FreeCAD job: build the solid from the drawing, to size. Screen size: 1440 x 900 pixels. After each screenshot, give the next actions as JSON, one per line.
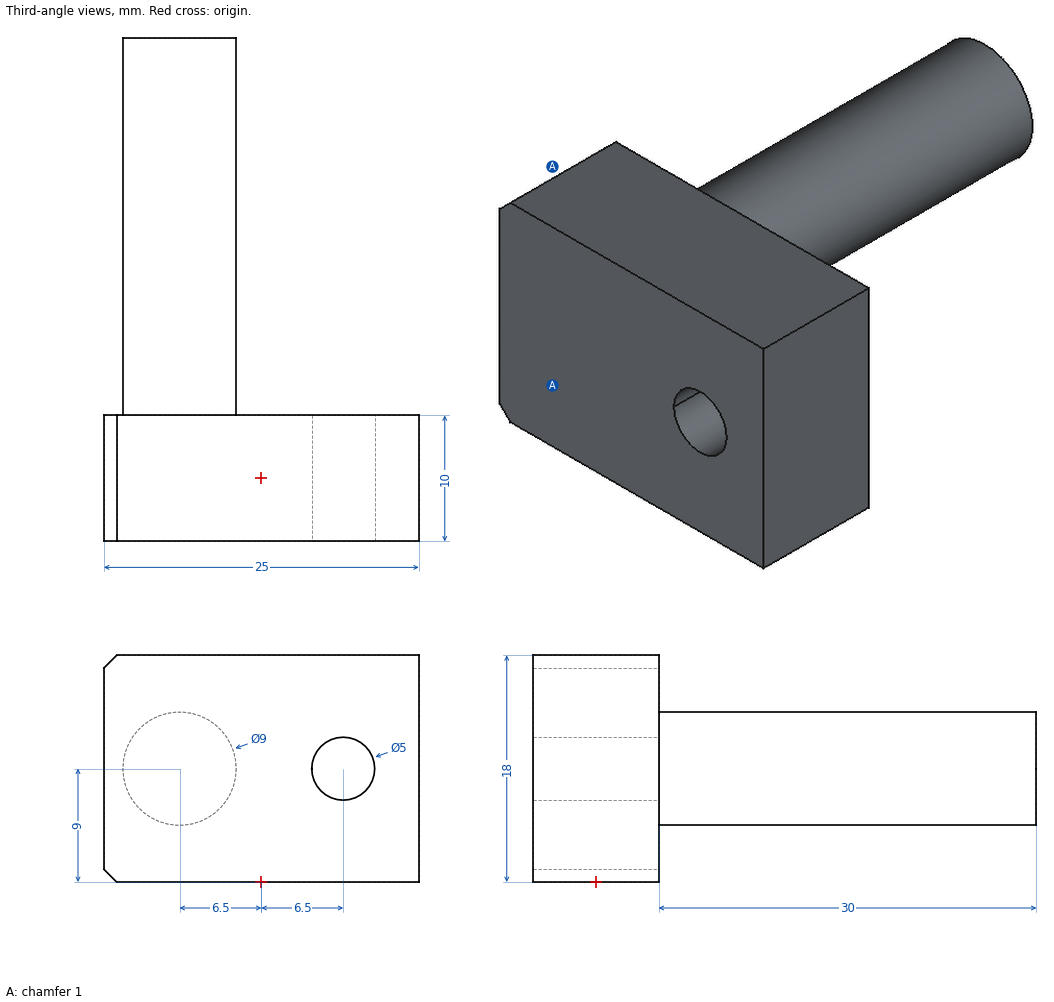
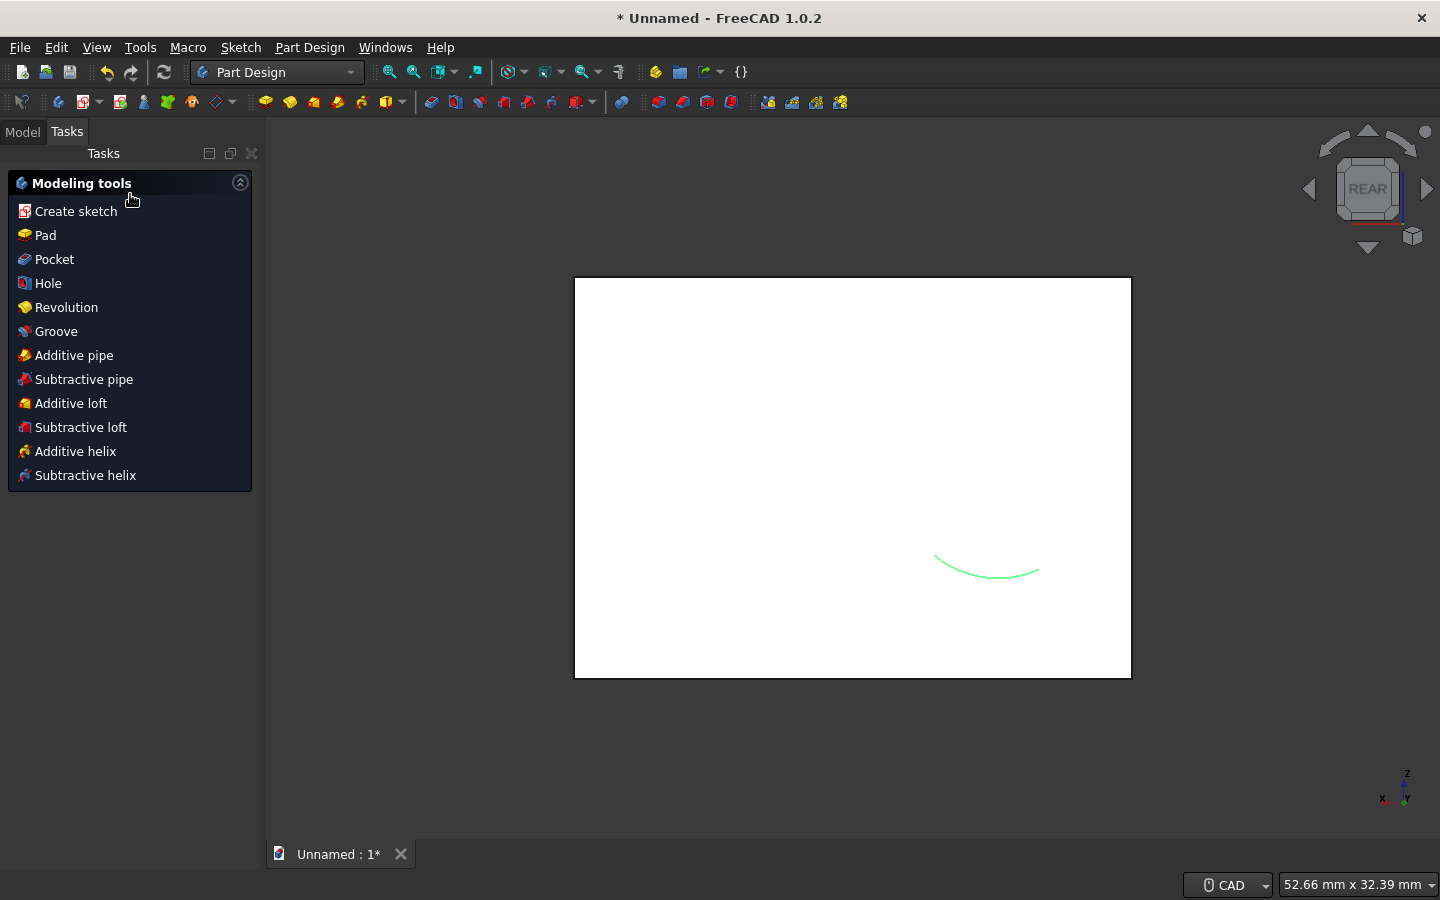
{"action": "left_click", "coordinate": [266, 102]}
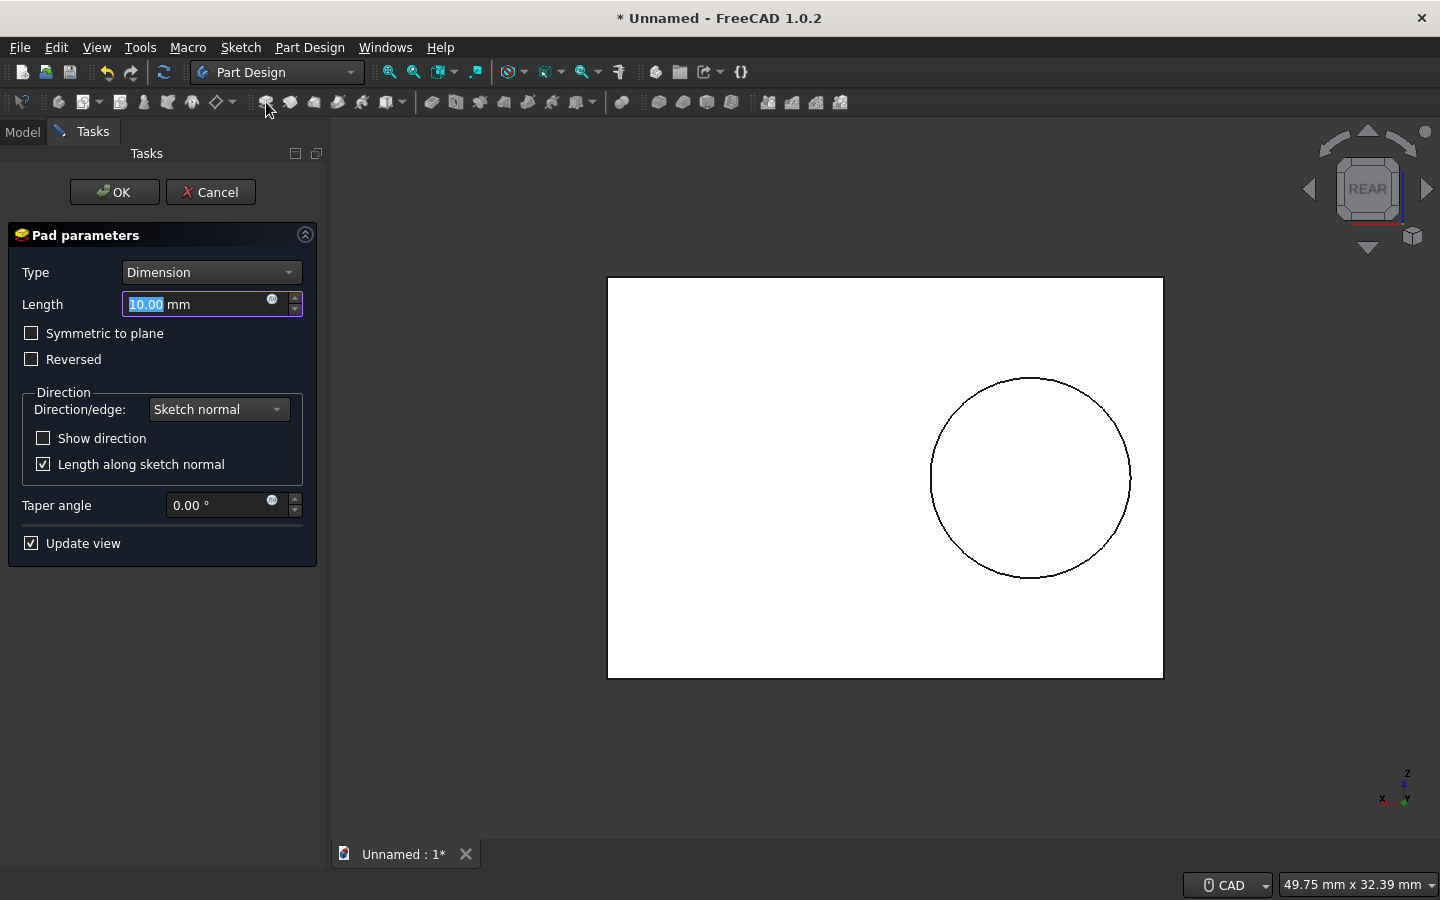
{"action": "type", "text": "30"}
{"action": "key", "text": "Tab"}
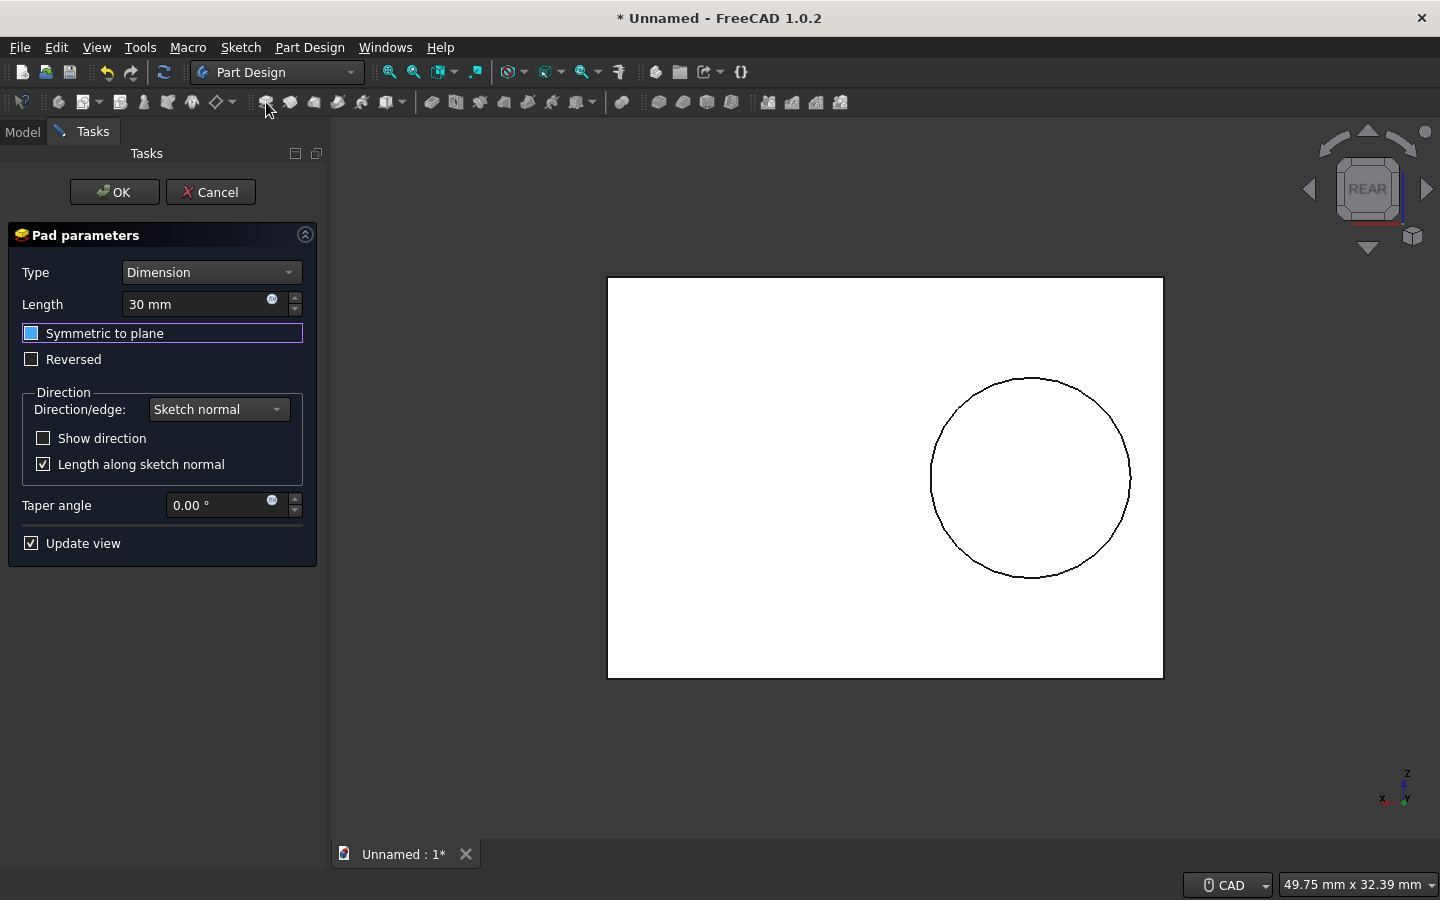
{"action": "left_click", "coordinate": [115, 192]}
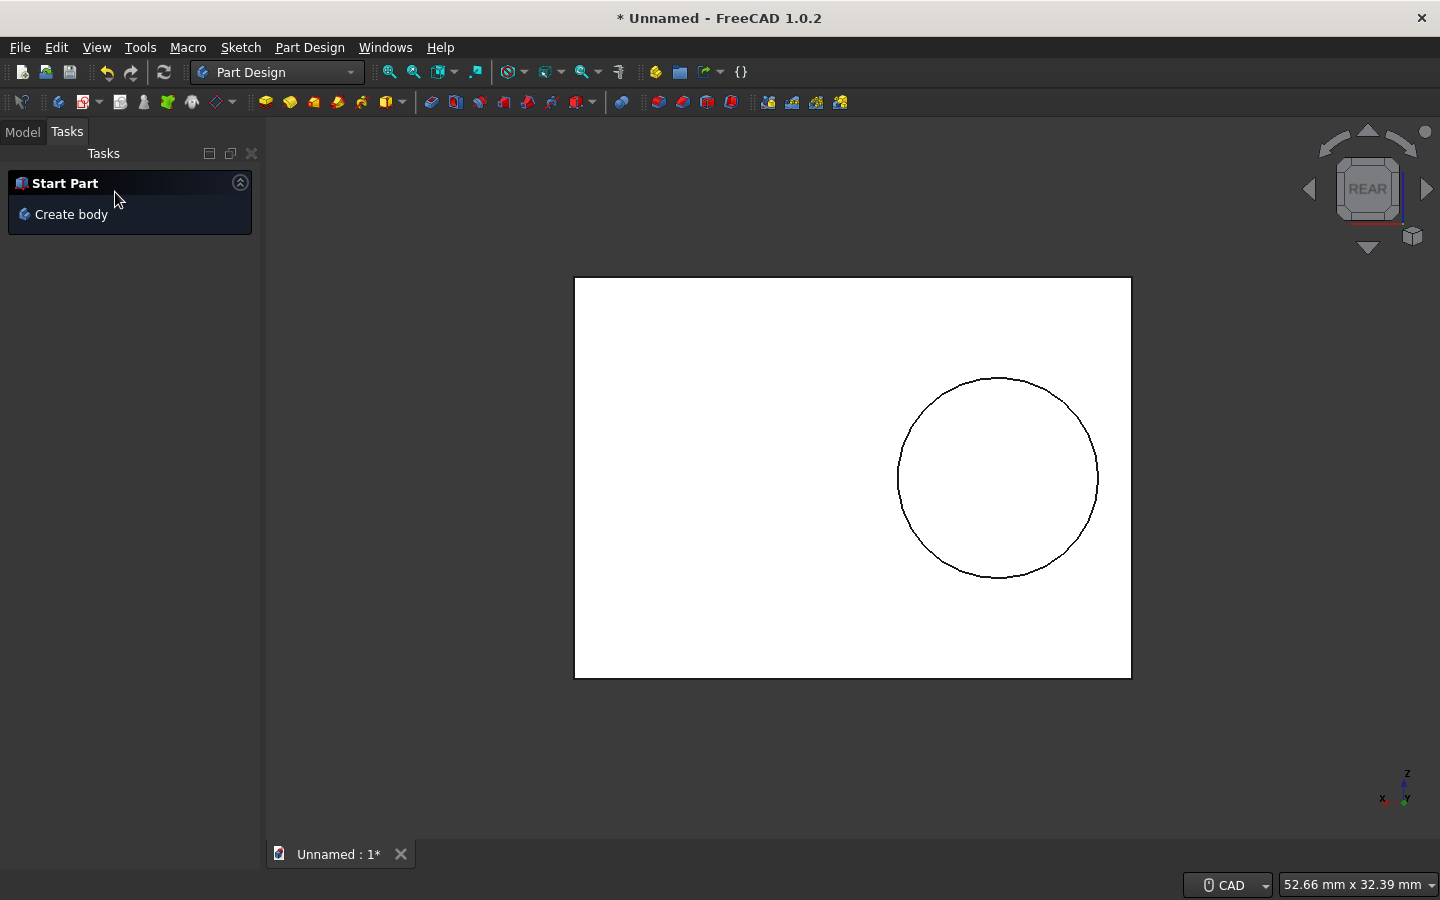
{"action": "left_click", "coordinate": [773, 534]}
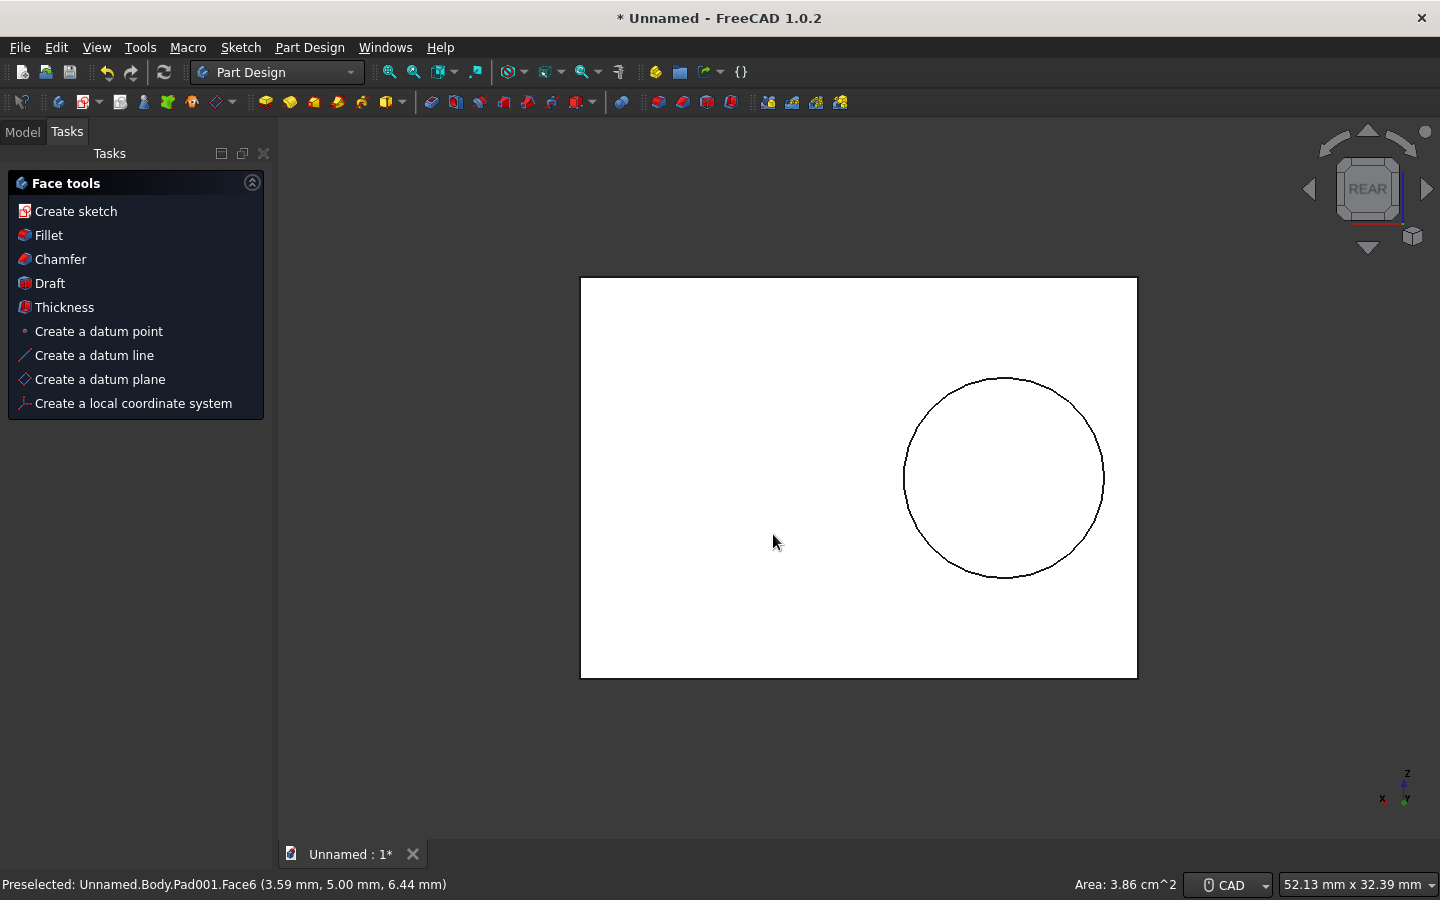
{"action": "left_click", "coordinate": [84, 102]}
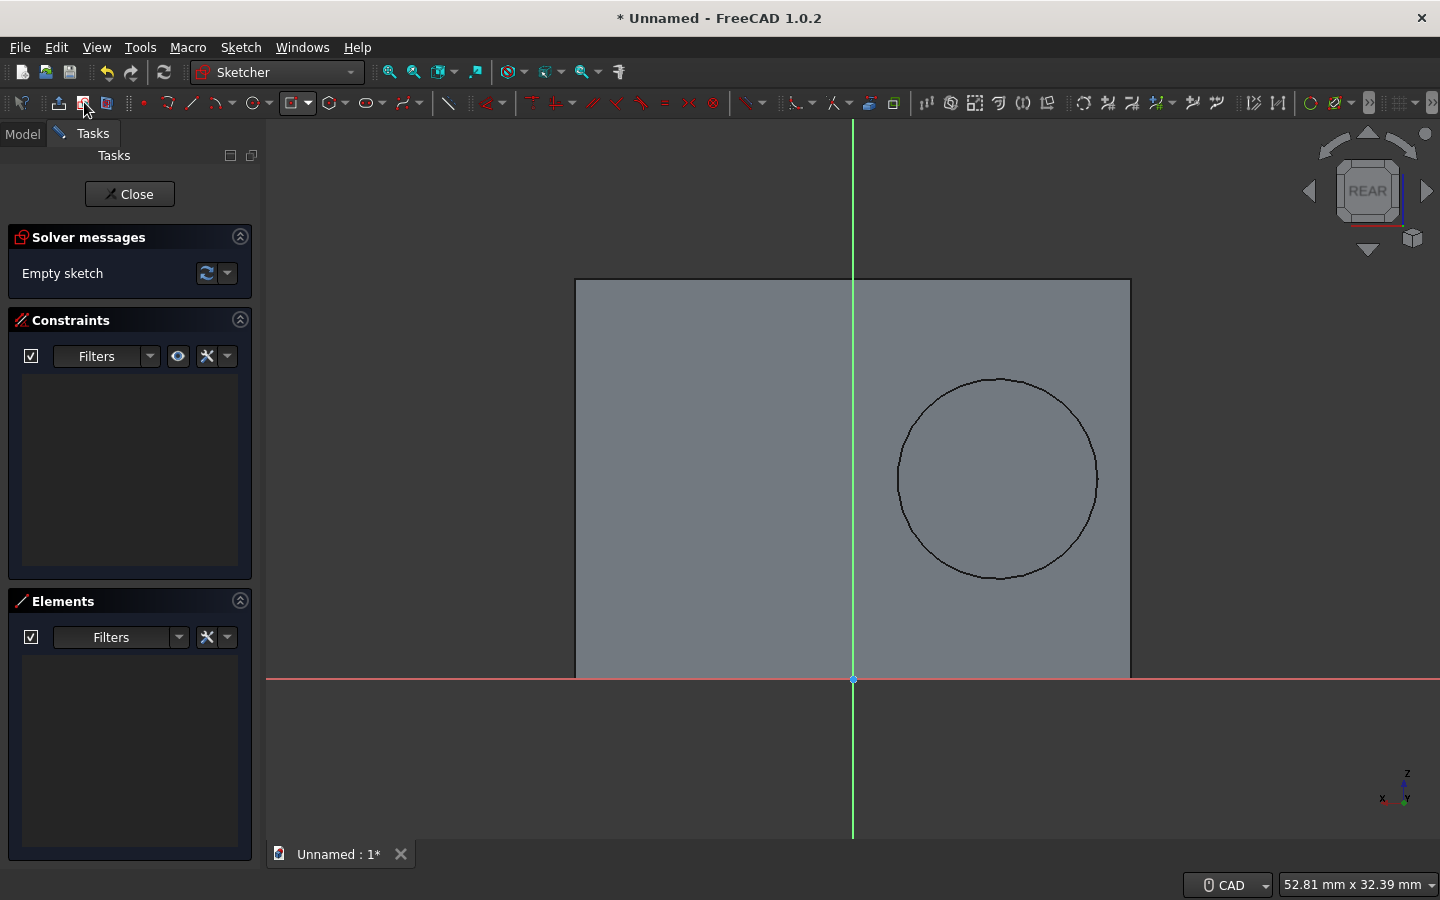
{"action": "key", "text": "q s"}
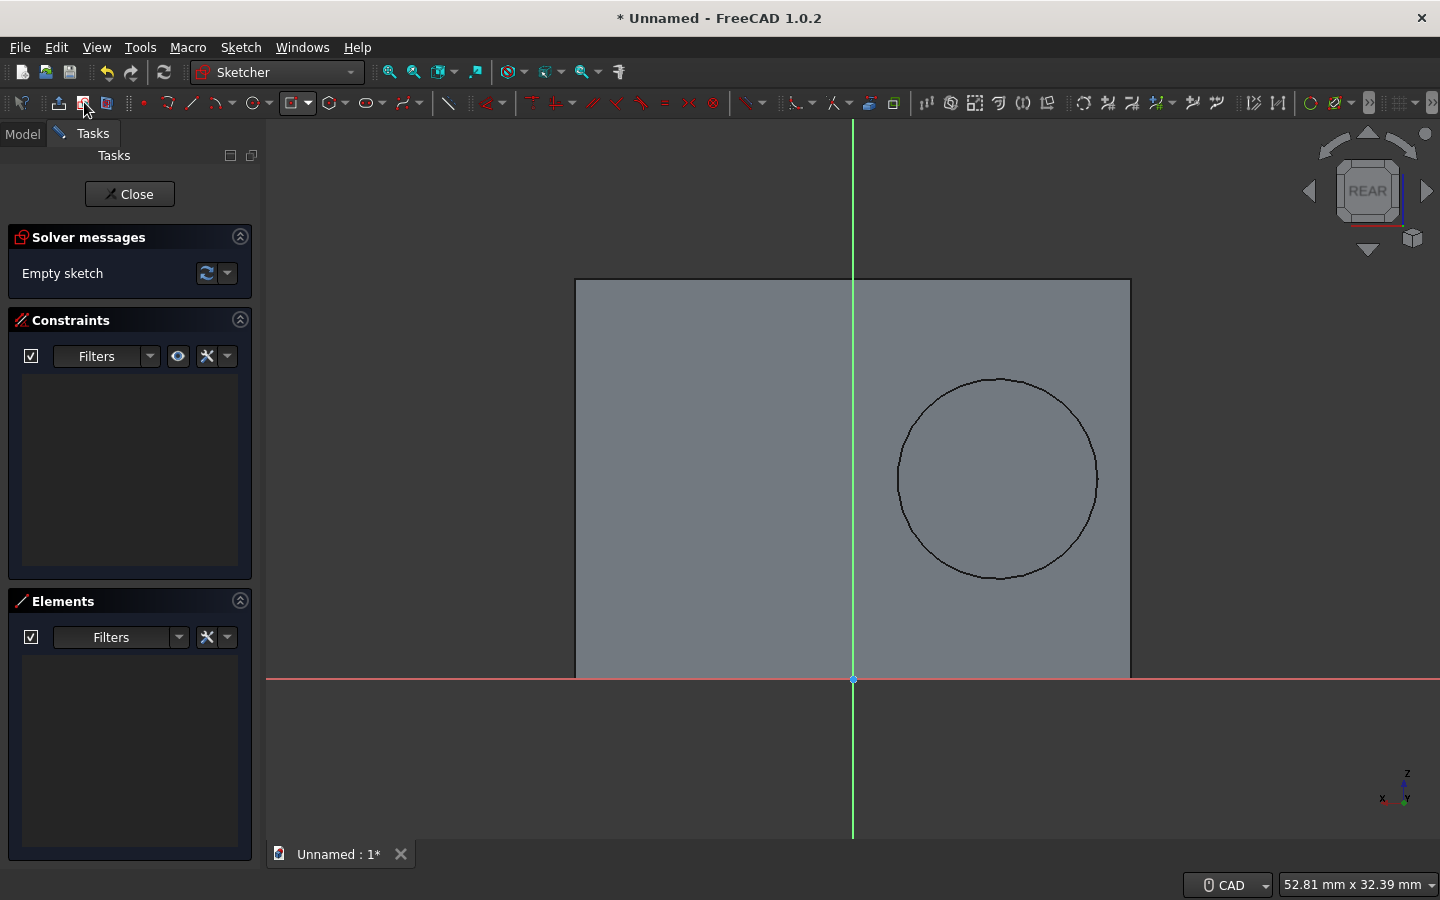
{"action": "scroll", "coordinate": [715, 639], "scroll_direction": "up", "scroll_amount": 3}